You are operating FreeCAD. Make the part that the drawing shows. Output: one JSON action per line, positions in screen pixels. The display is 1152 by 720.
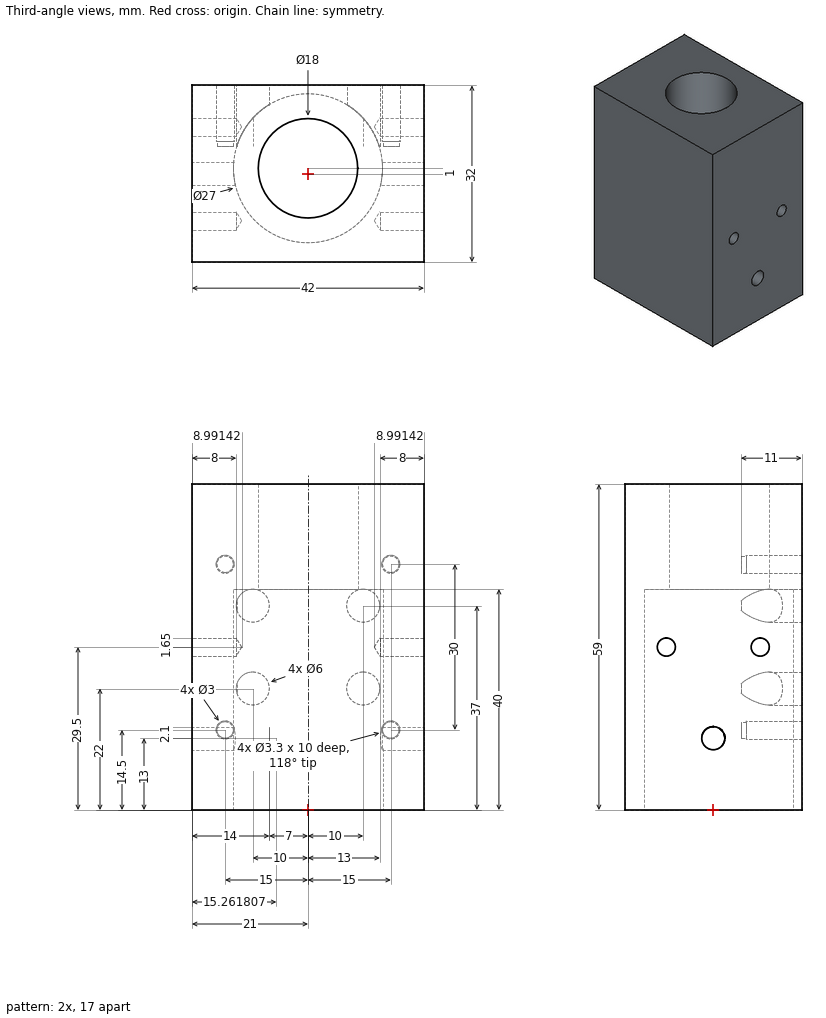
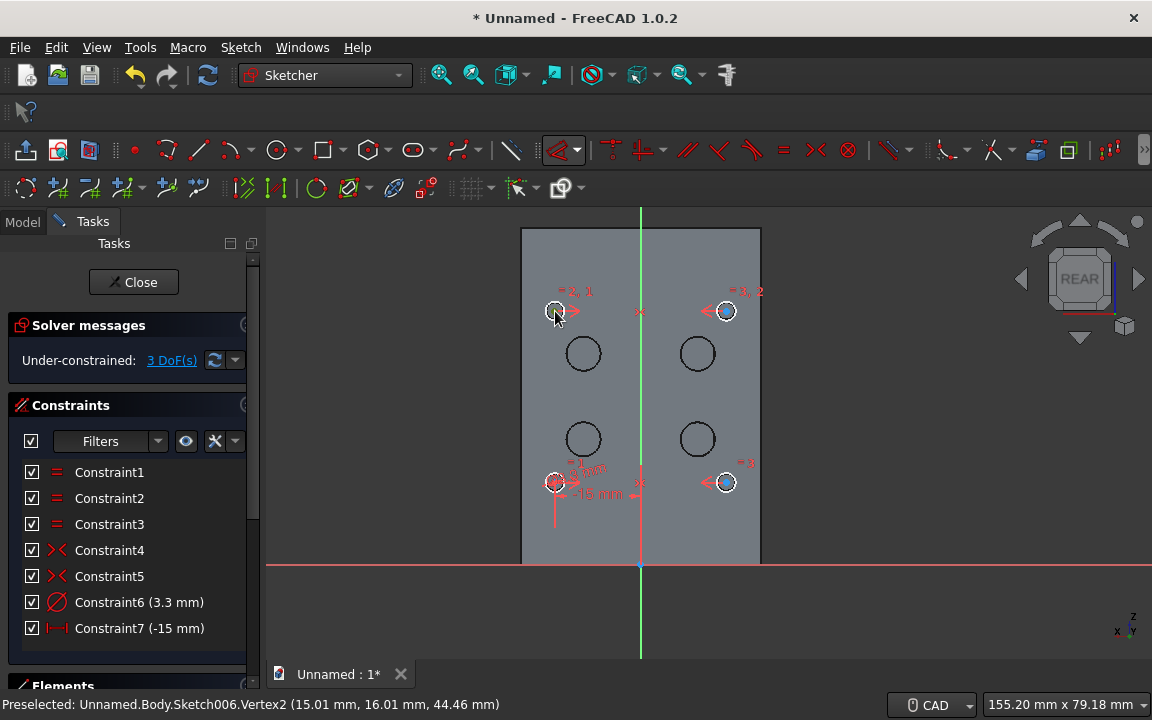
{"action": "key", "text": "l"}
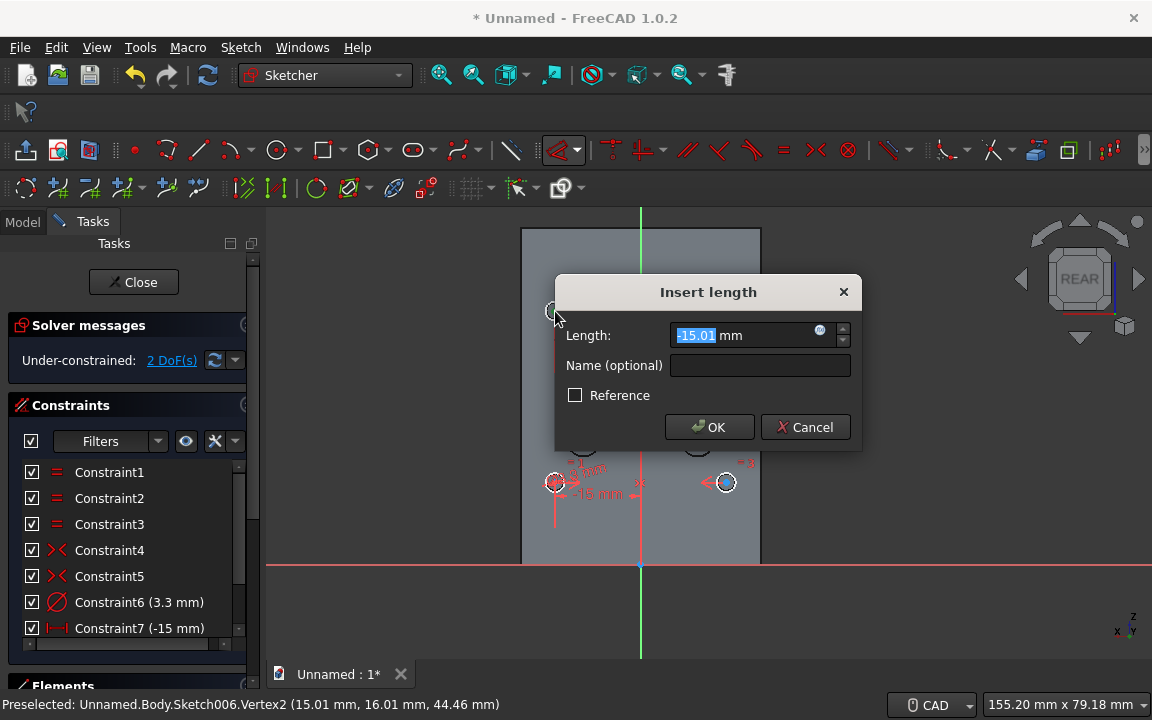
{"action": "type", "text": "-15"}
{"action": "key", "text": "Return"}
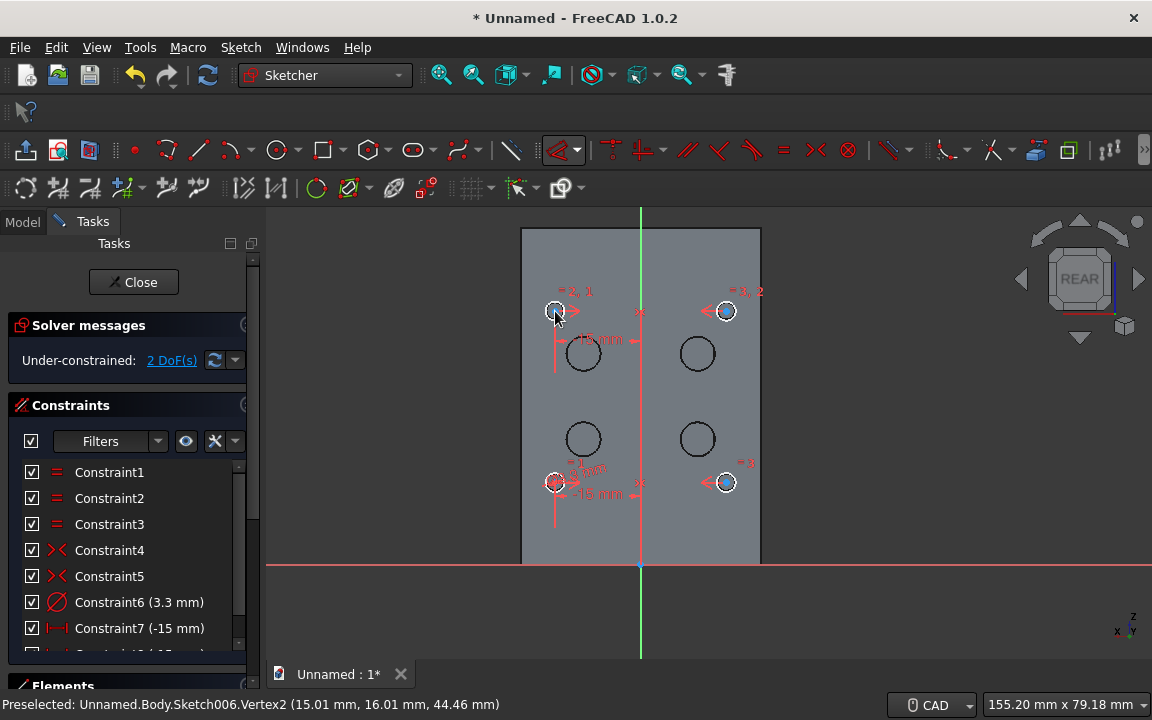
{"action": "left_click", "coordinate": [555, 483]}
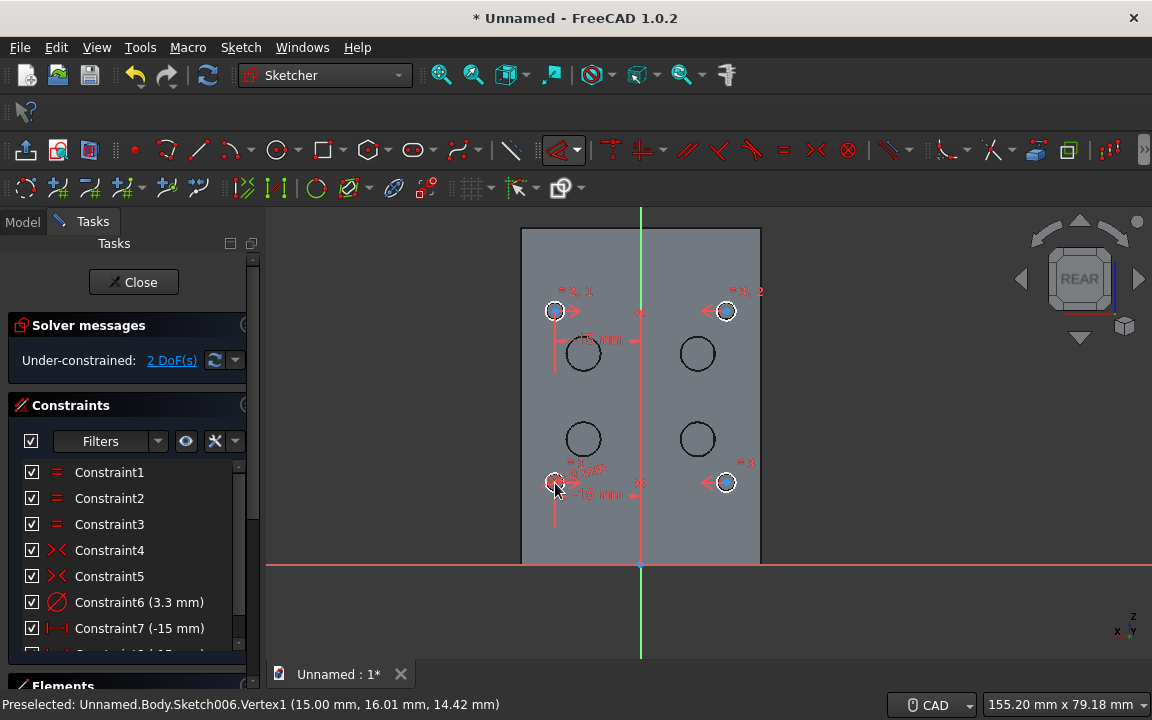
{"action": "left_click", "coordinate": [555, 311]}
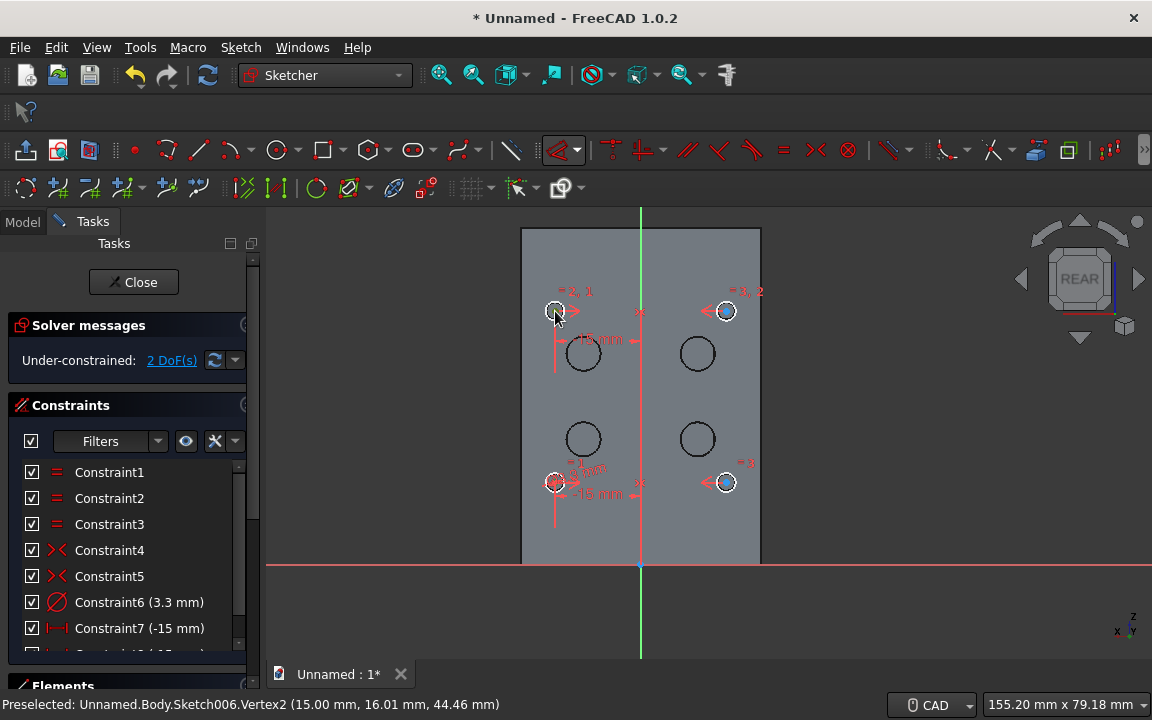
{"action": "key", "text": "i"}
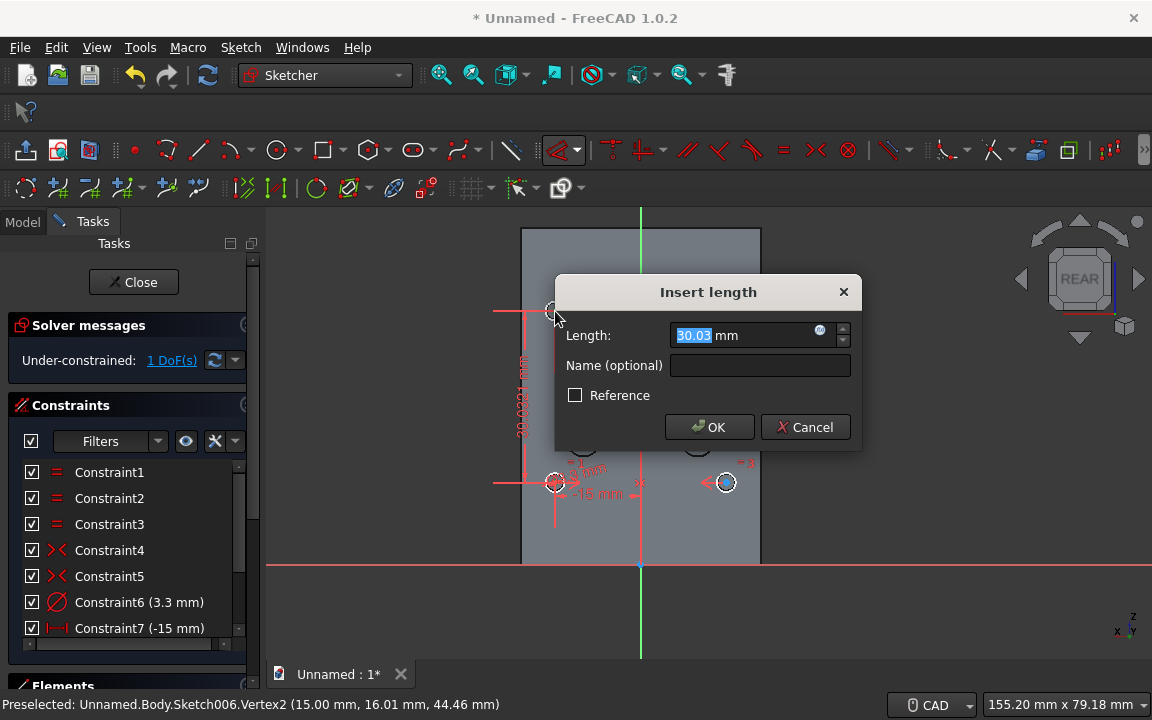
{"action": "type", "text": "30"}
{"action": "key", "text": "Return"}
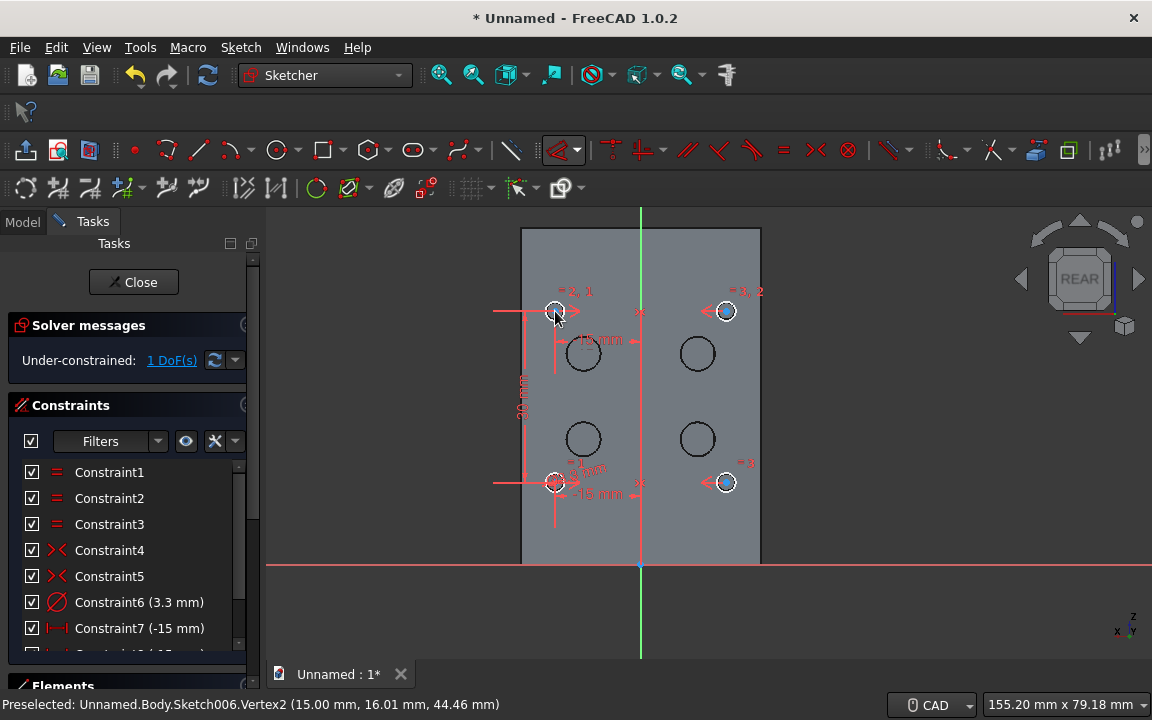
{"action": "left_click", "coordinate": [555, 483]}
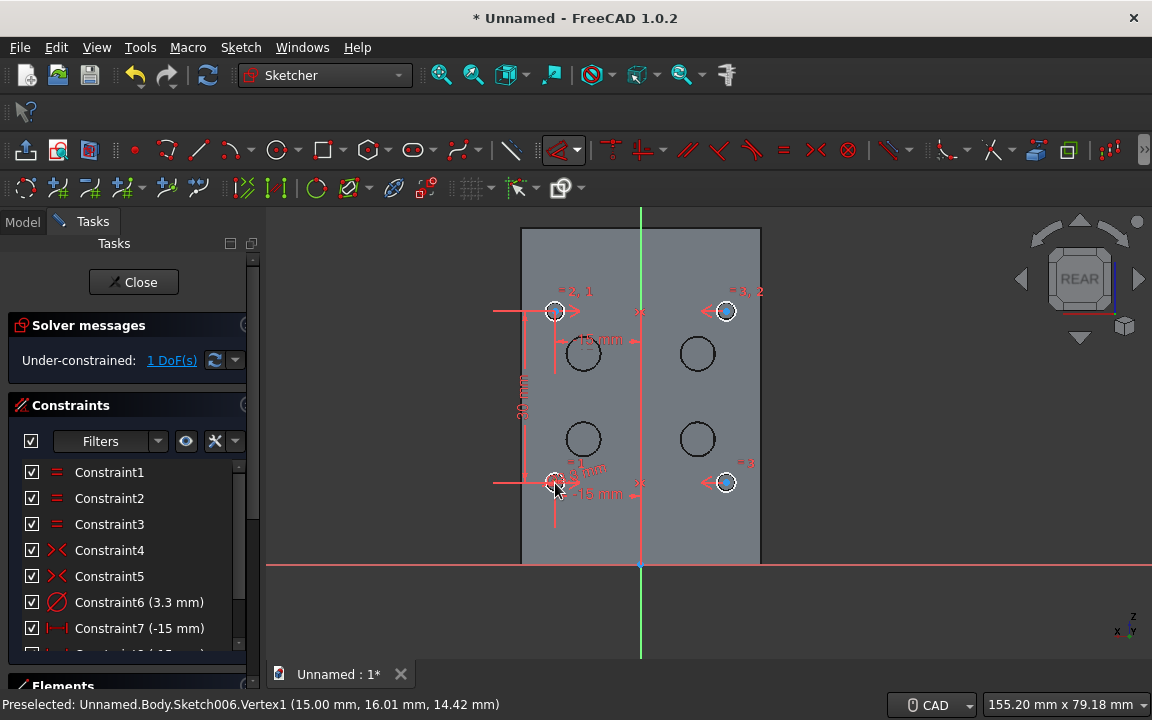
{"action": "key", "text": "i"}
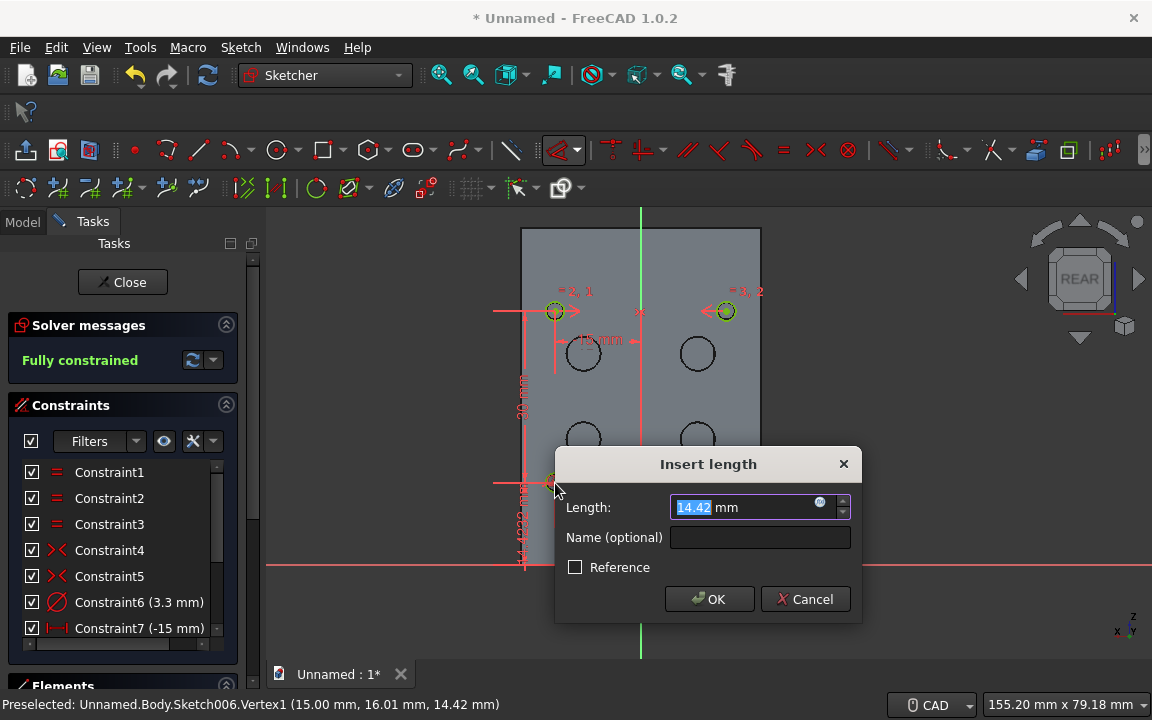
{"action": "type", "text": "14.5"}
{"action": "key", "text": "Return"}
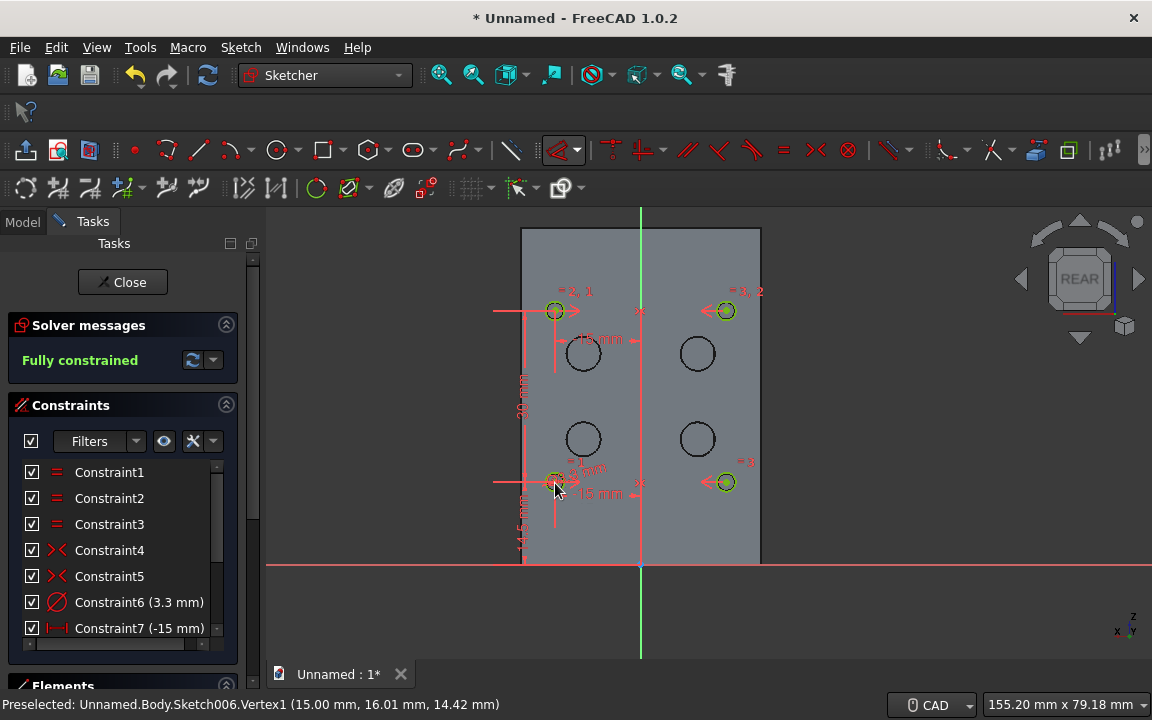
{"action": "left_click", "coordinate": [123, 282]}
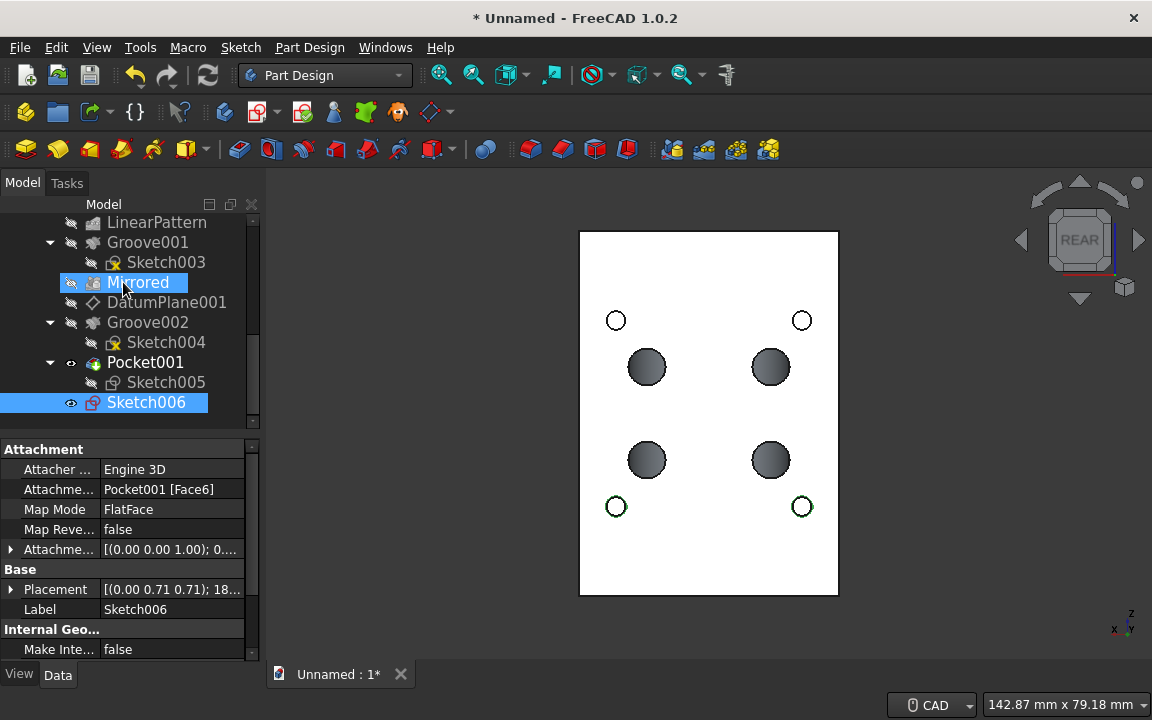
{"action": "left_click", "coordinate": [272, 150]}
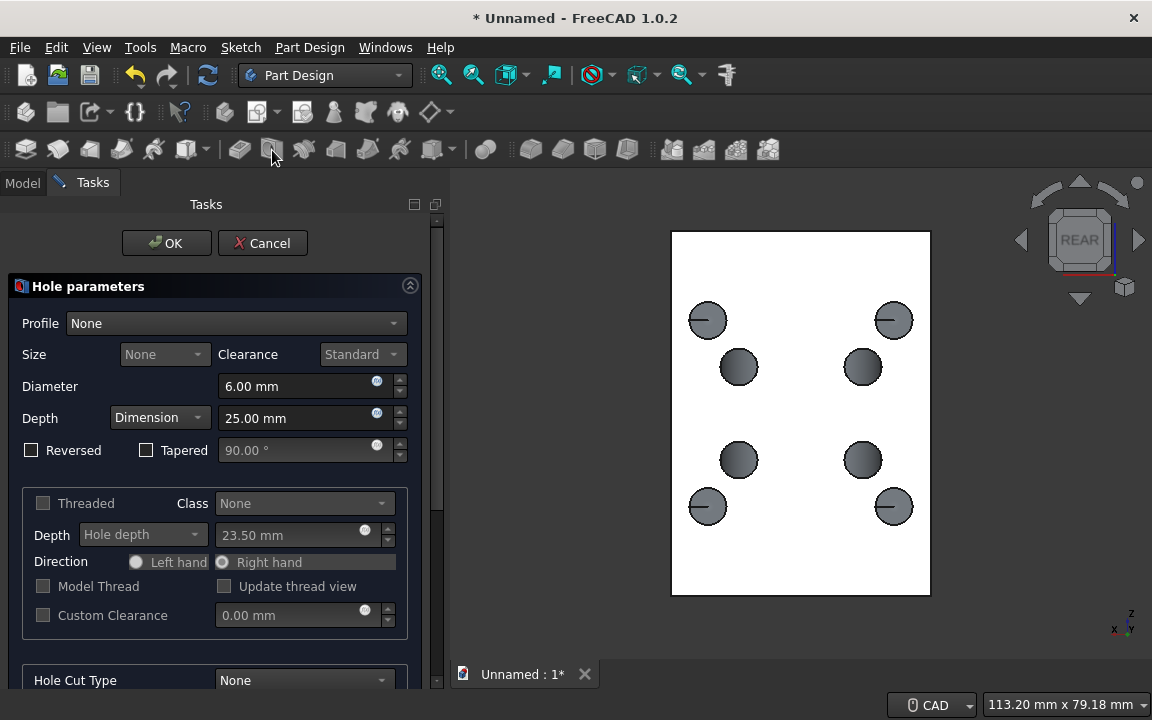
{"action": "triple_click", "coordinate": [305, 386]}